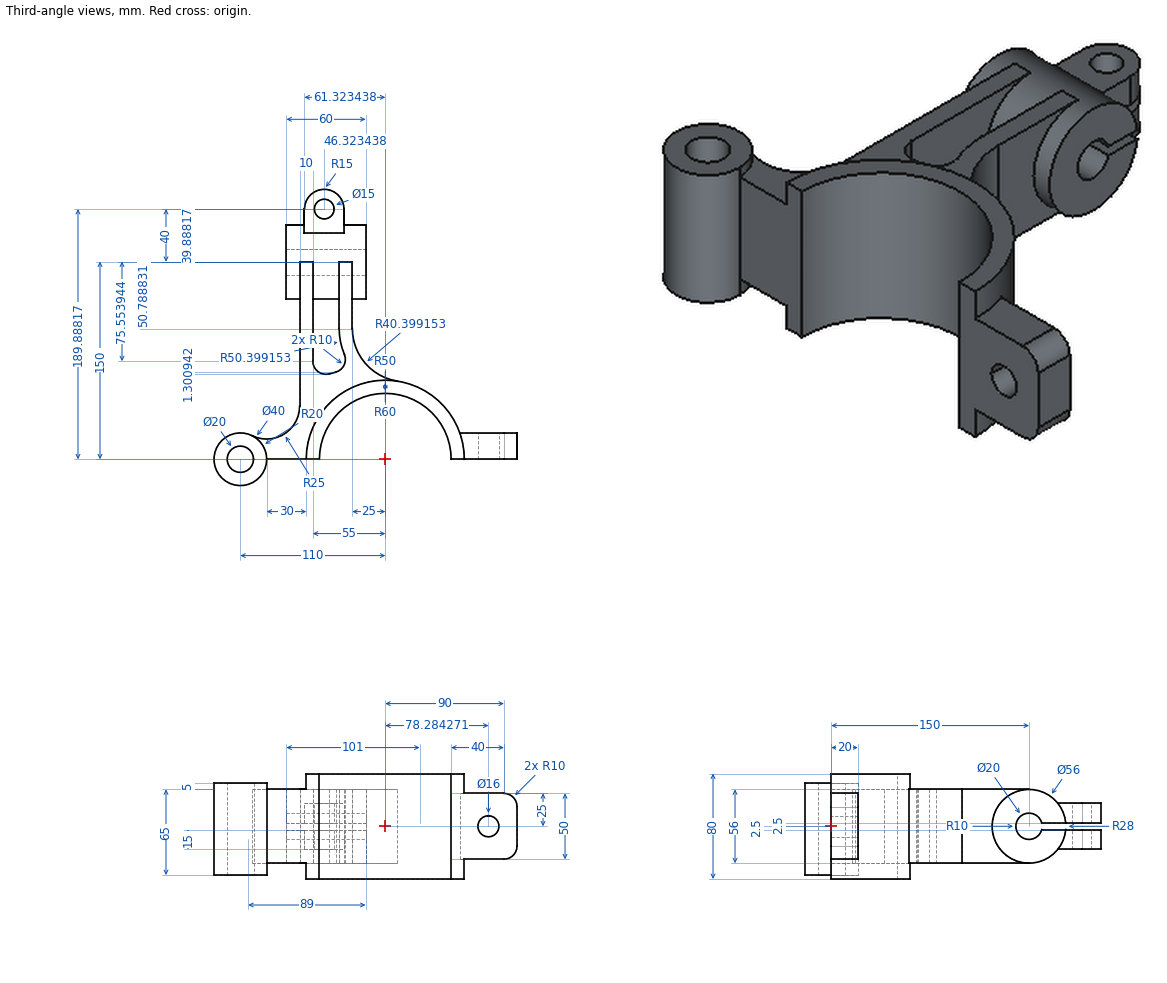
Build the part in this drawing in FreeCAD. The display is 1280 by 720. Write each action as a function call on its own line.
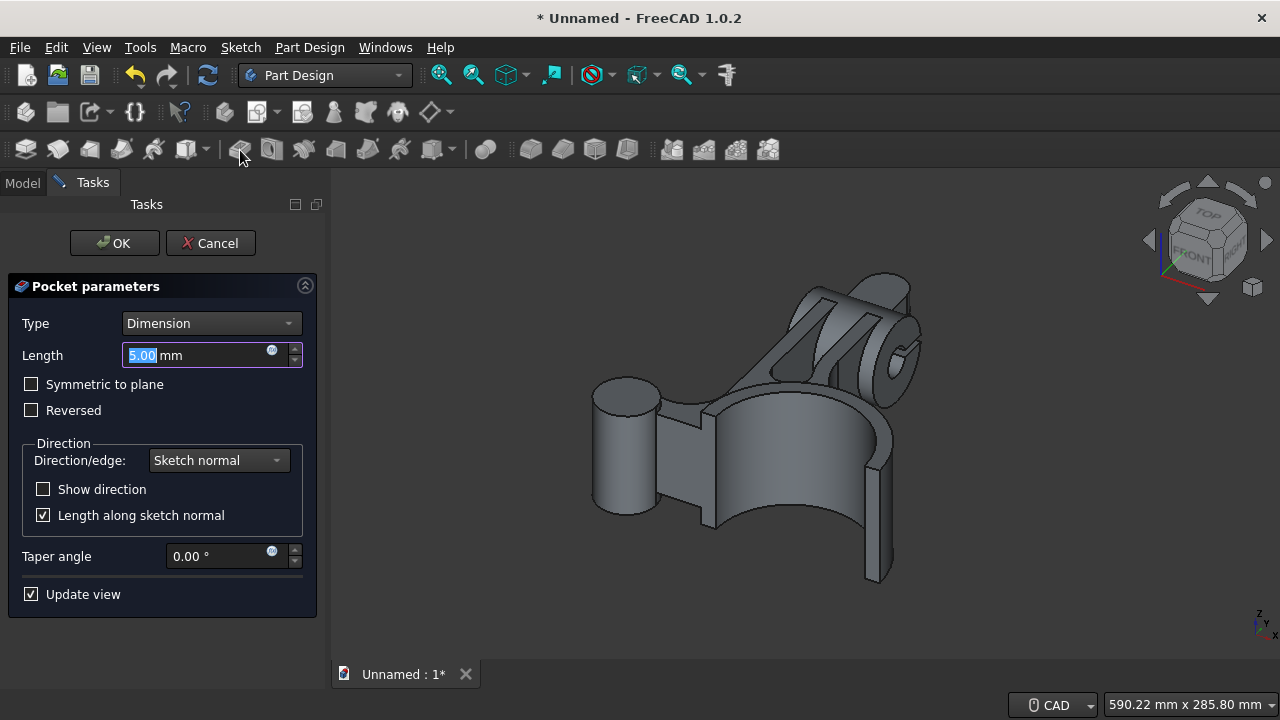
text(89)
key(Tab)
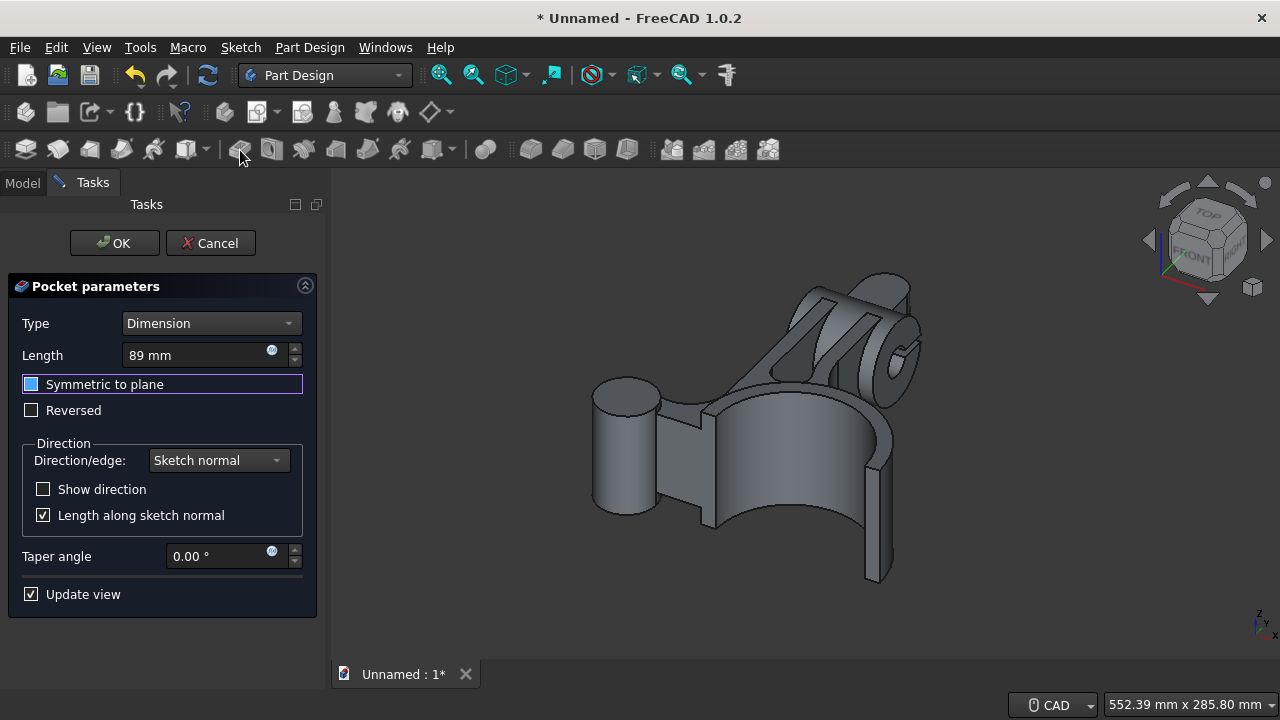
click(115, 243)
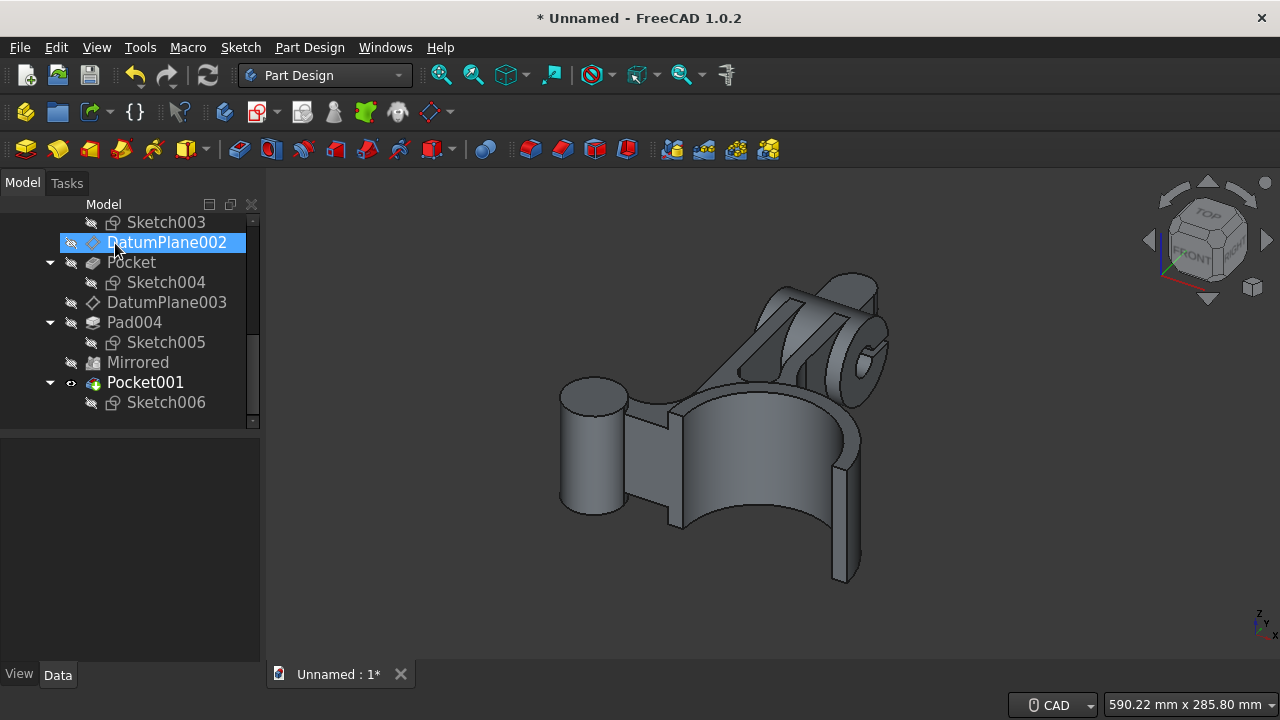
click(851, 288)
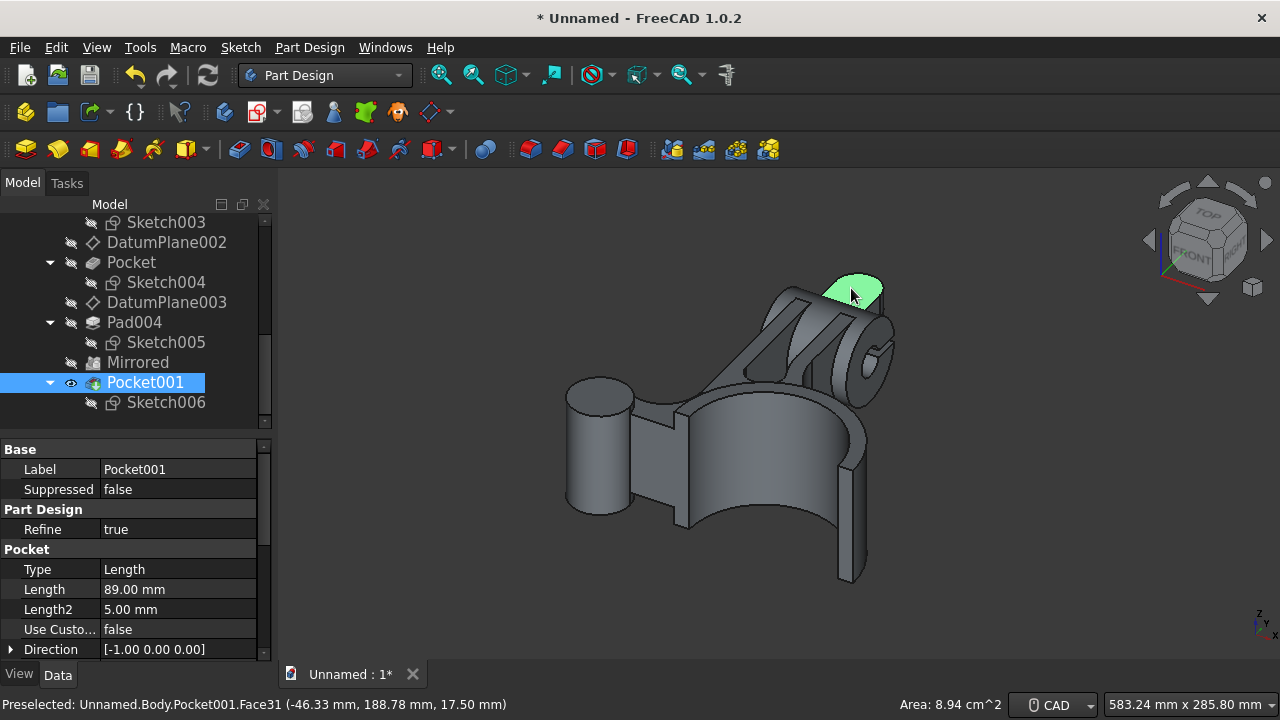
click(258, 112)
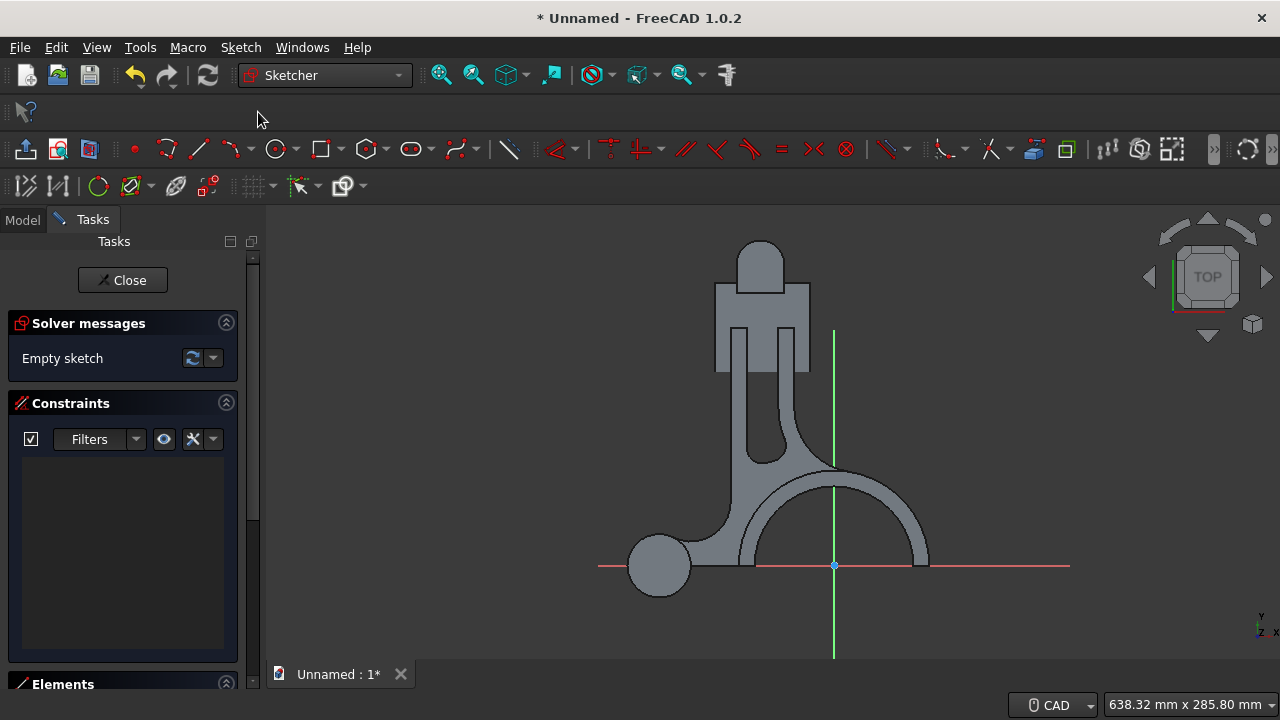
scroll(766, 247, up, 12)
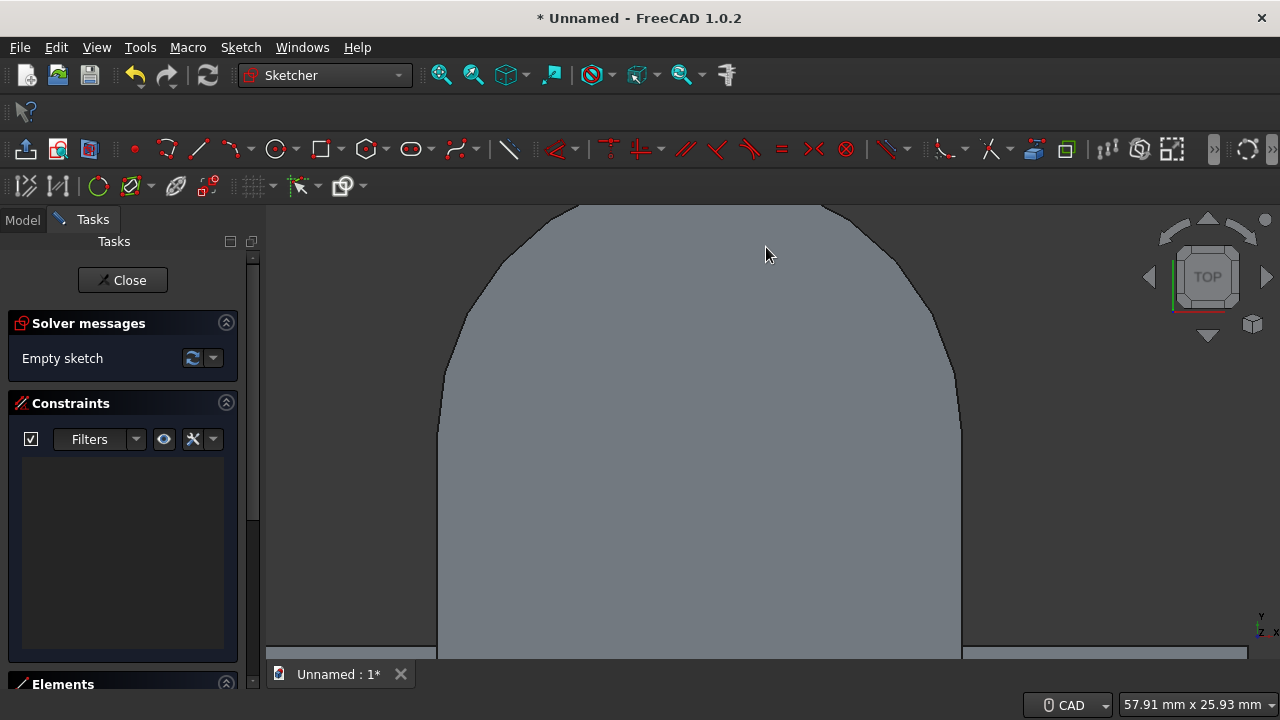
key(g)
key(c)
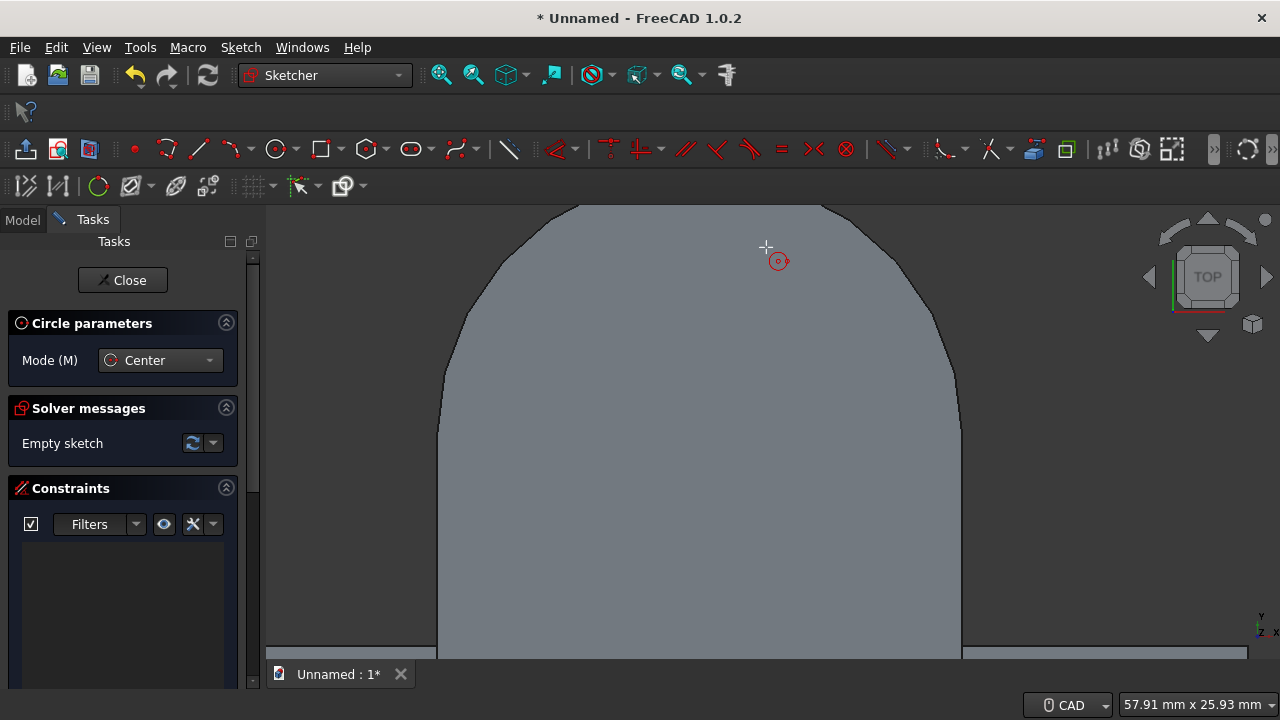
click(700, 436)
move(793, 343)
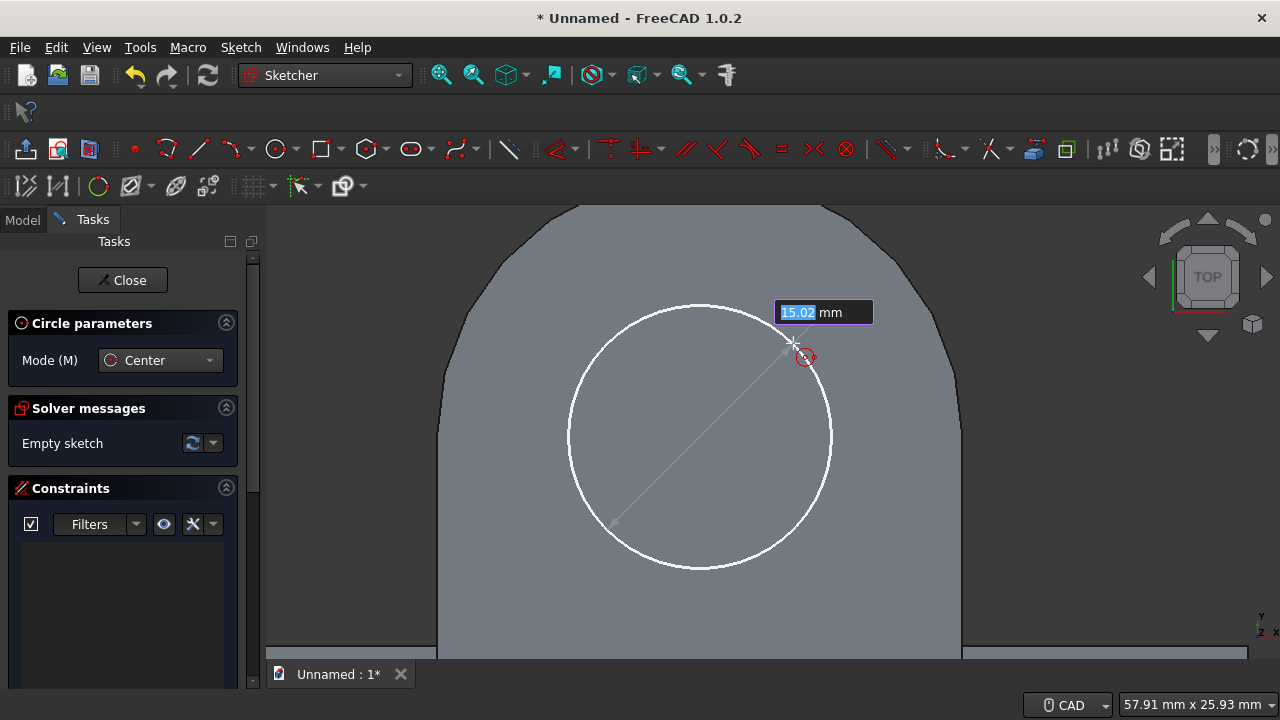
text(15)
key(Return)
key(Escape)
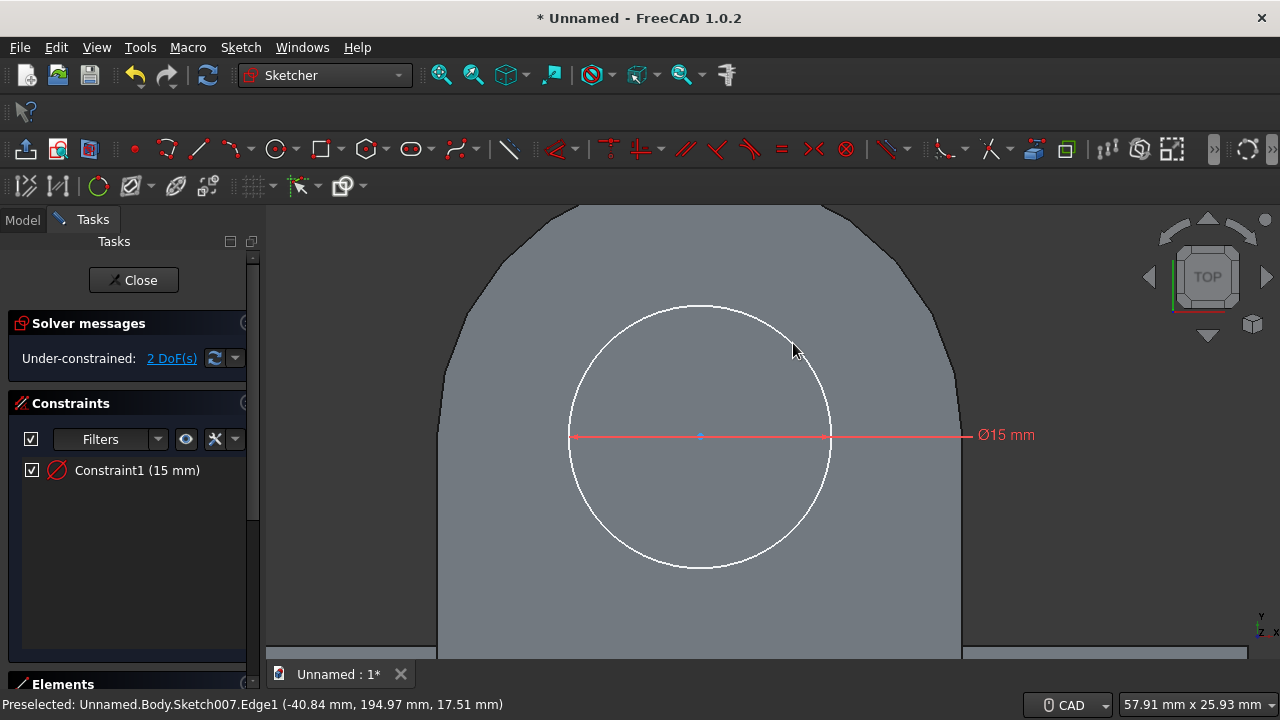
key(d)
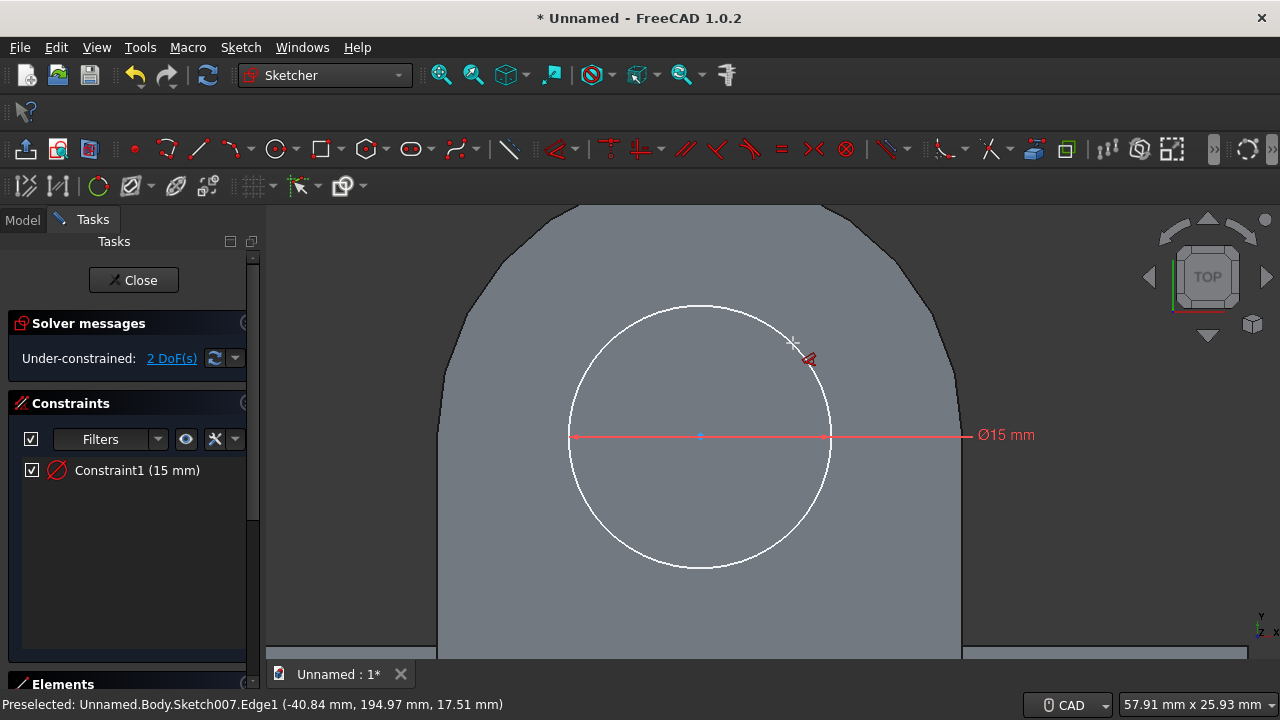
click(700, 437)
click(908, 403)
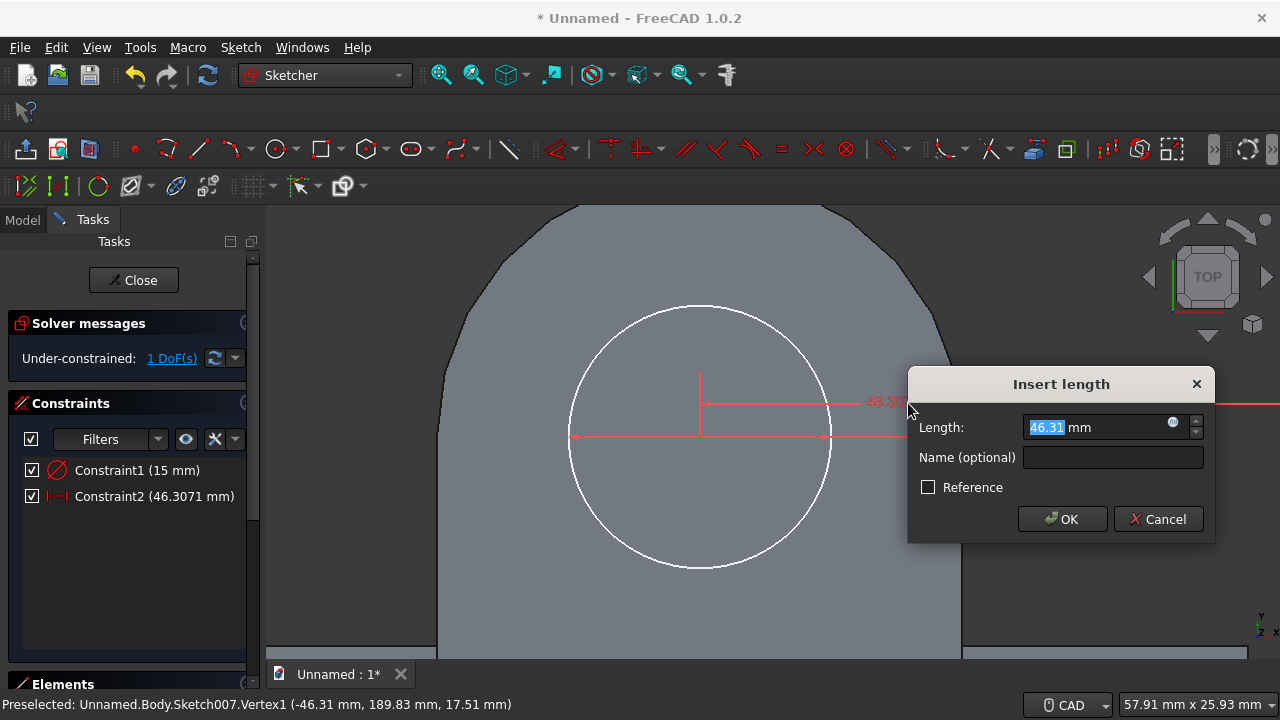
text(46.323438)
key(Return)